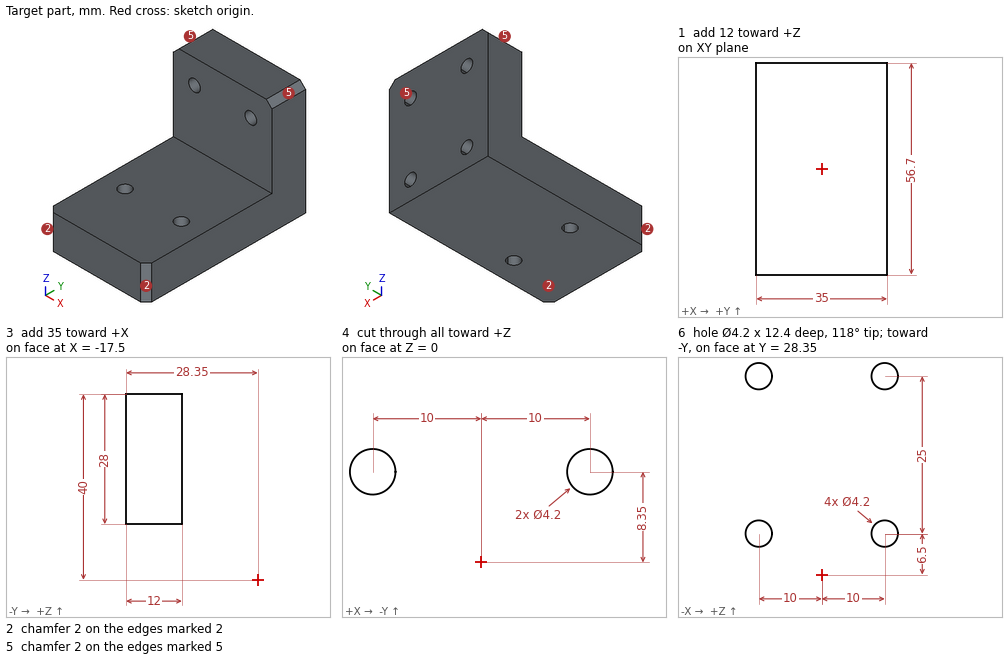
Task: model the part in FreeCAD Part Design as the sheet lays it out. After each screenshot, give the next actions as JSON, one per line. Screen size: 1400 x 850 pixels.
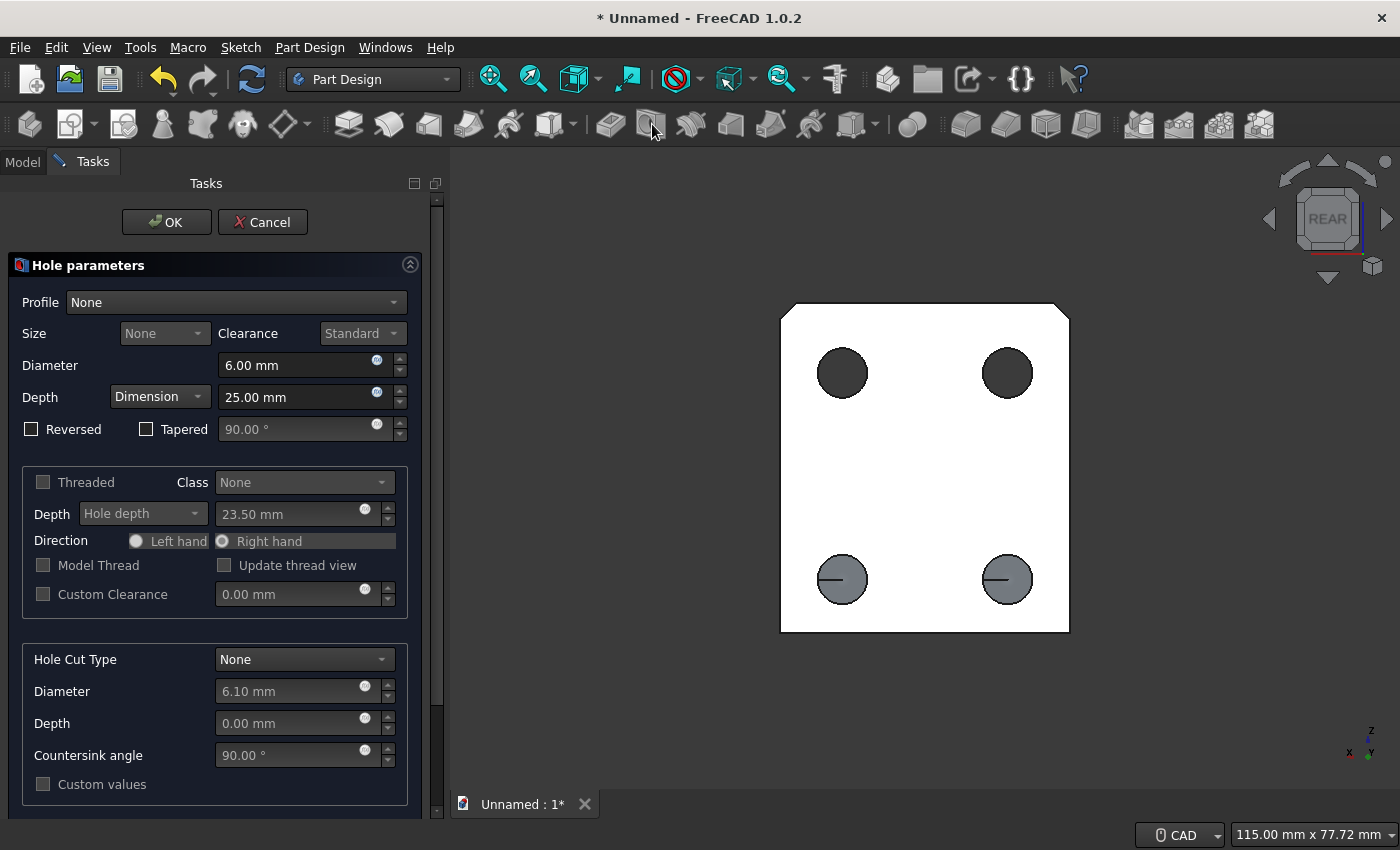
{"action": "triple_click", "coordinate": [305, 365]}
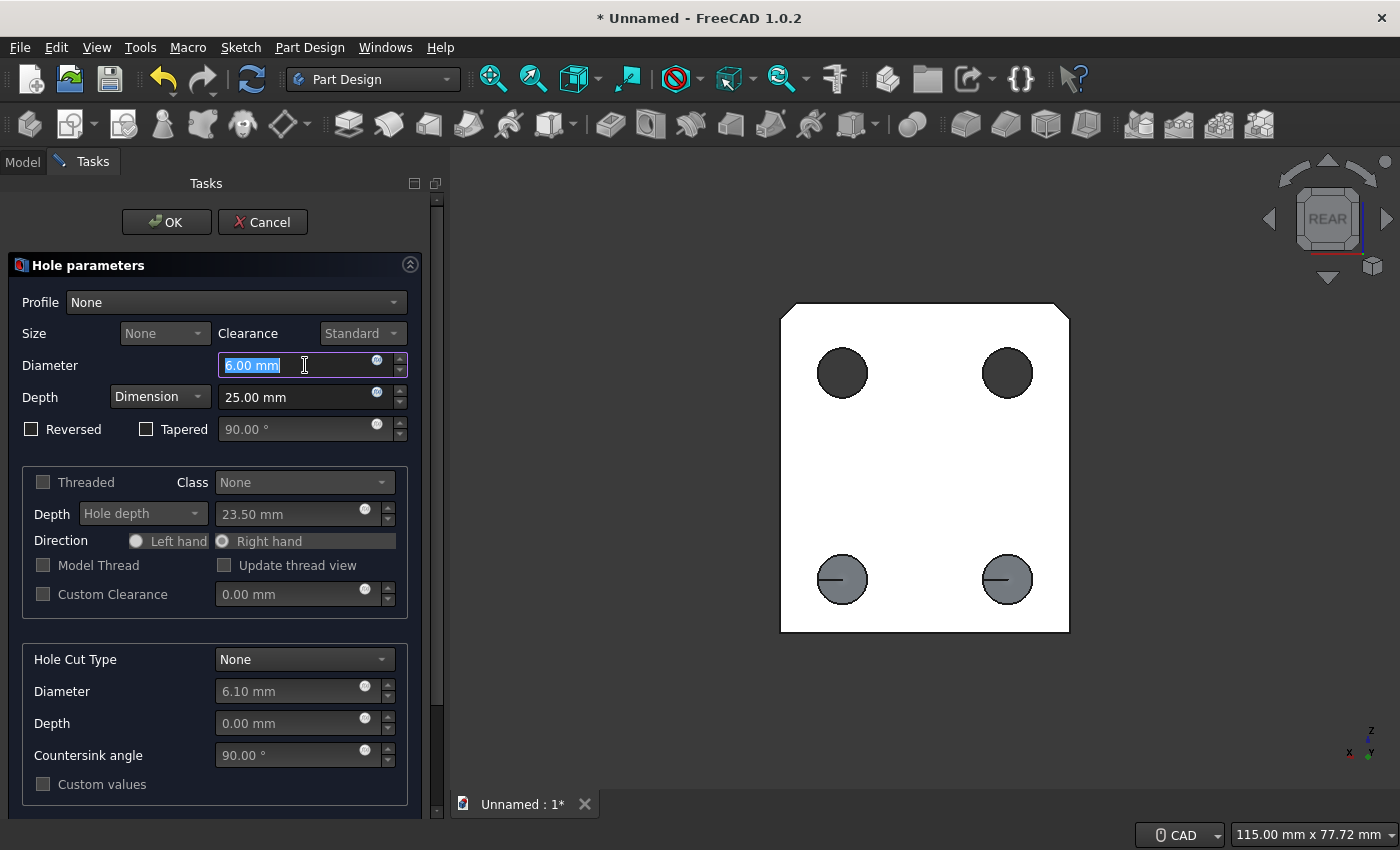
{"action": "type", "text": "4.2"}
{"action": "key", "text": "Tab"}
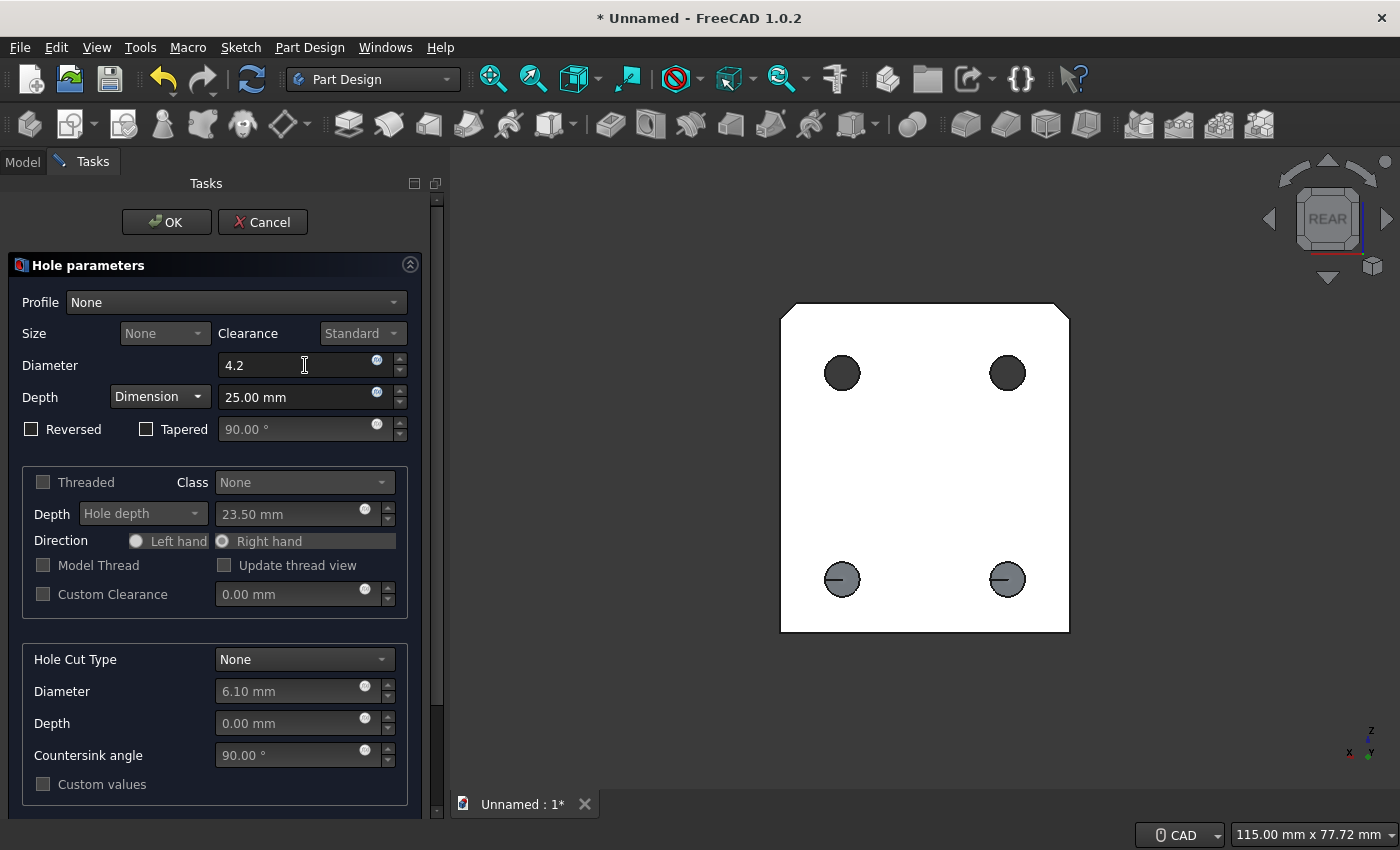
{"action": "triple_click", "coordinate": [305, 397]}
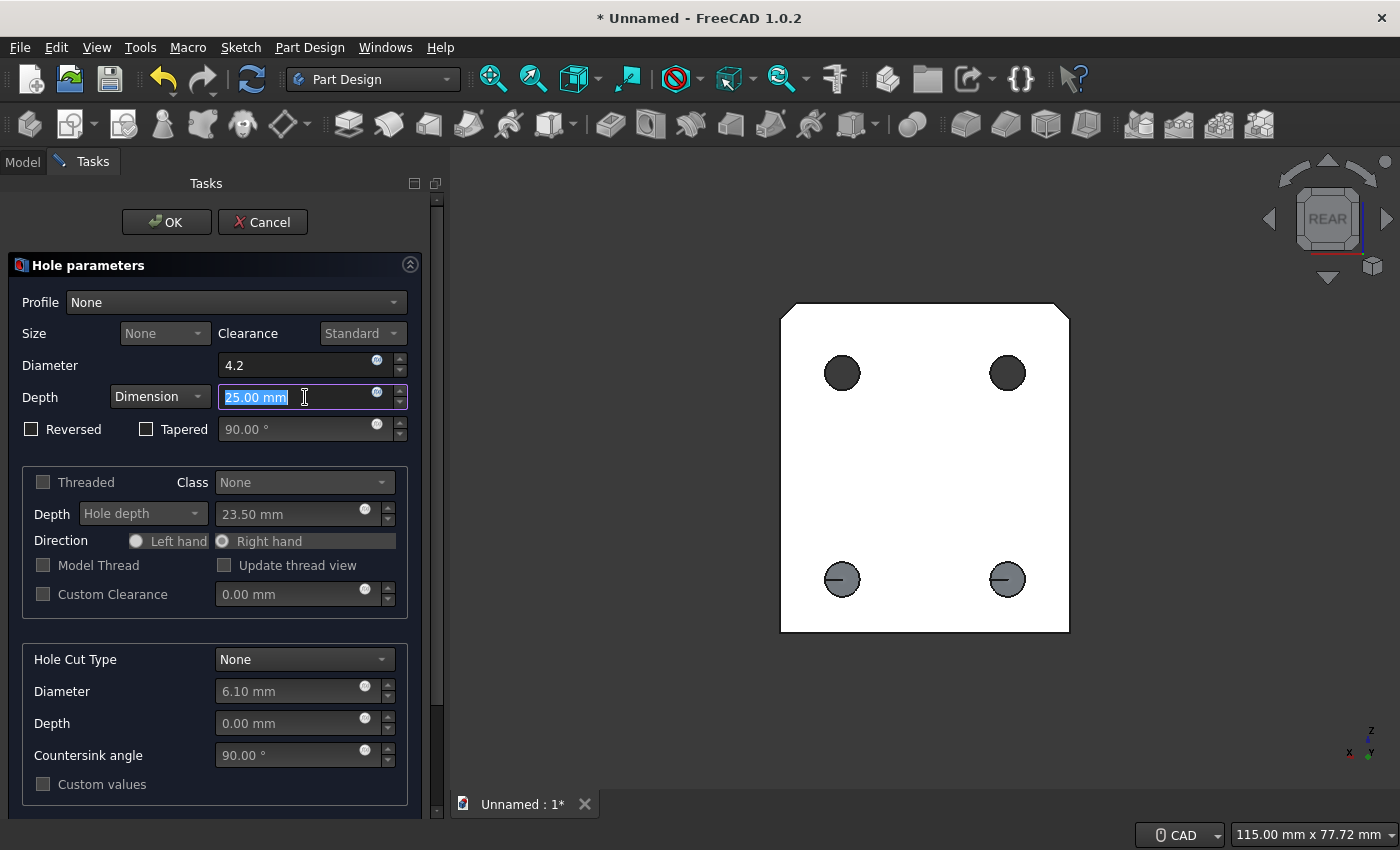
{"action": "type", "text": "12.4"}
{"action": "key", "text": "Tab"}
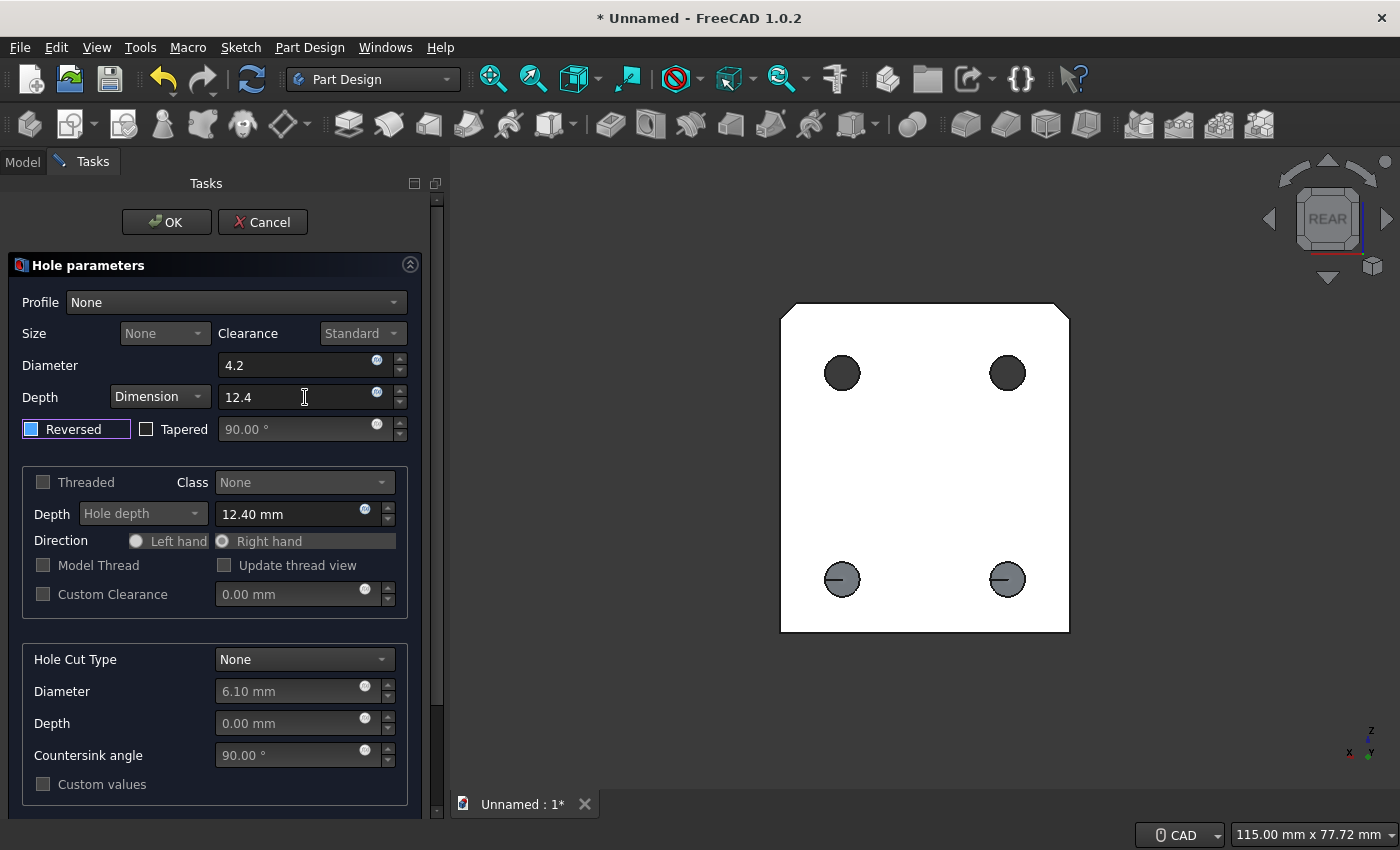
{"action": "left_click", "coordinate": [167, 222]}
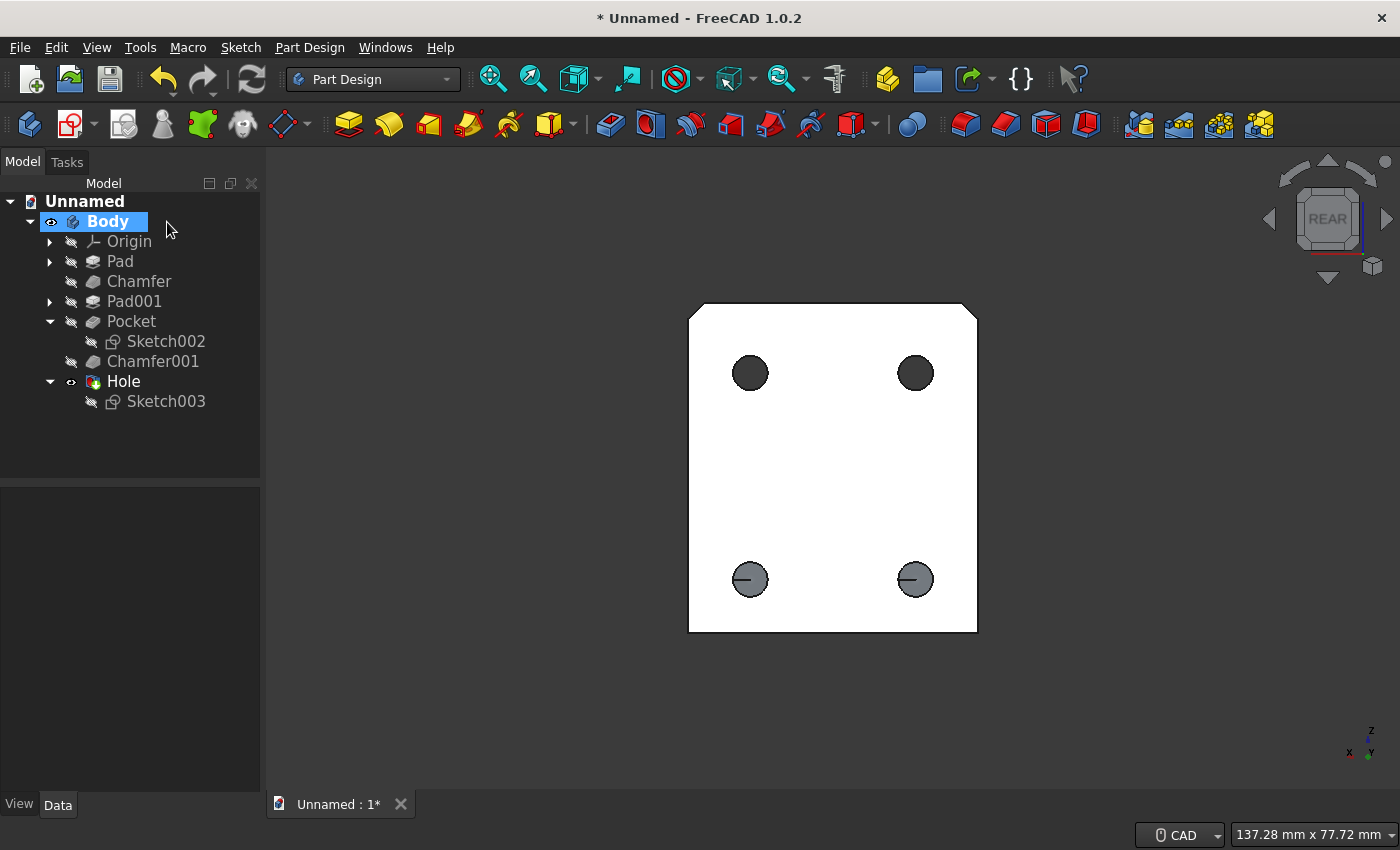
{"action": "key", "text": "0"}